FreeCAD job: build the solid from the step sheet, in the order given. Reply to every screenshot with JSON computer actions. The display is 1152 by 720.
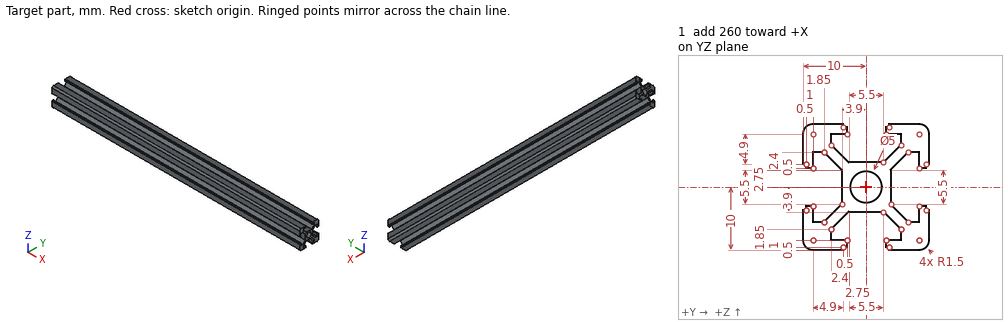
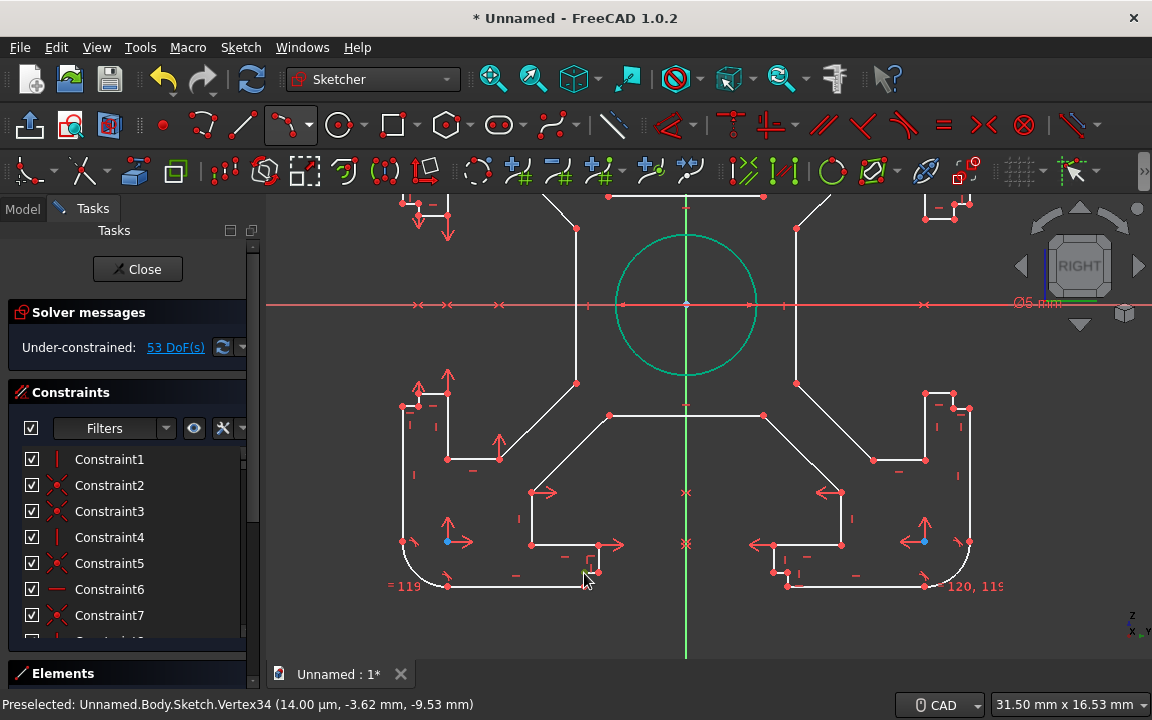
{"action": "left_click", "coordinate": [788, 573]}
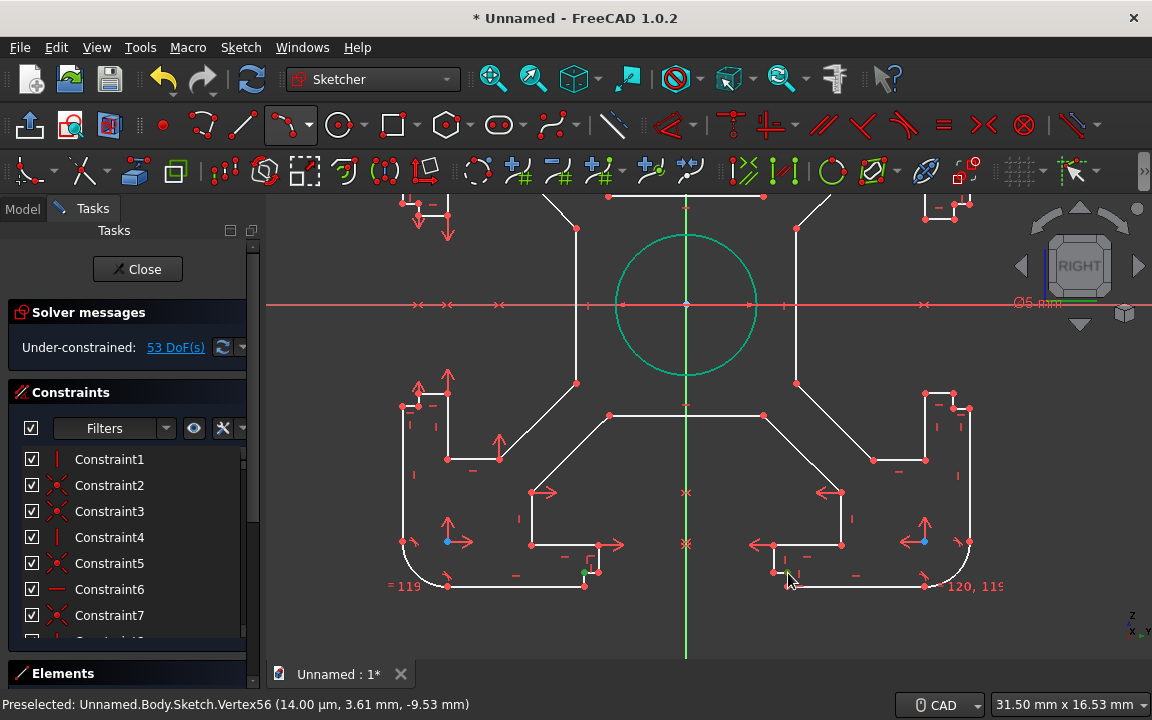
{"action": "left_click", "coordinate": [686, 602]}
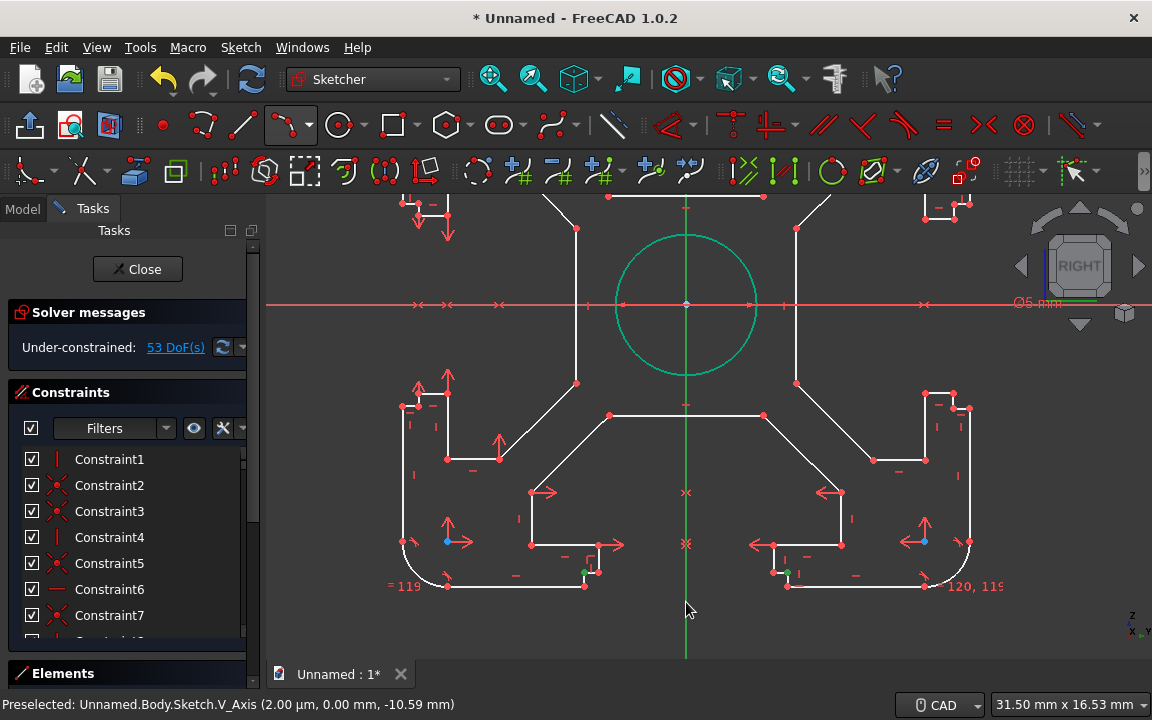
{"action": "key", "text": "s"}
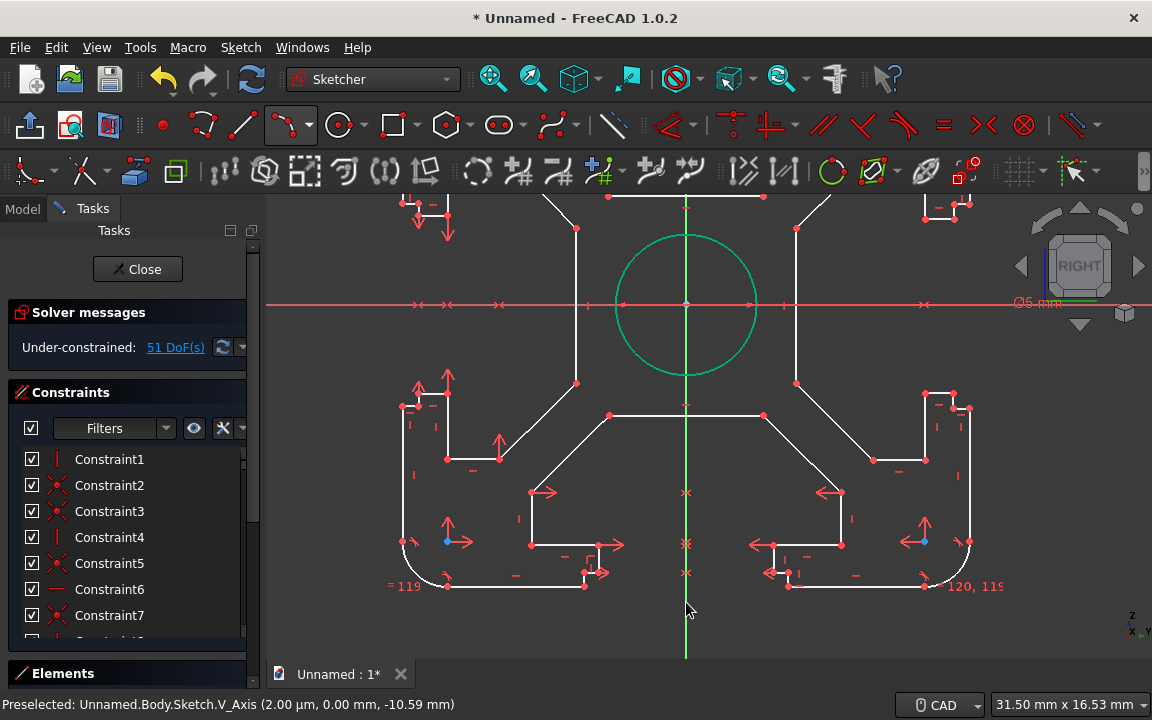
{"action": "left_click", "coordinate": [419, 406]}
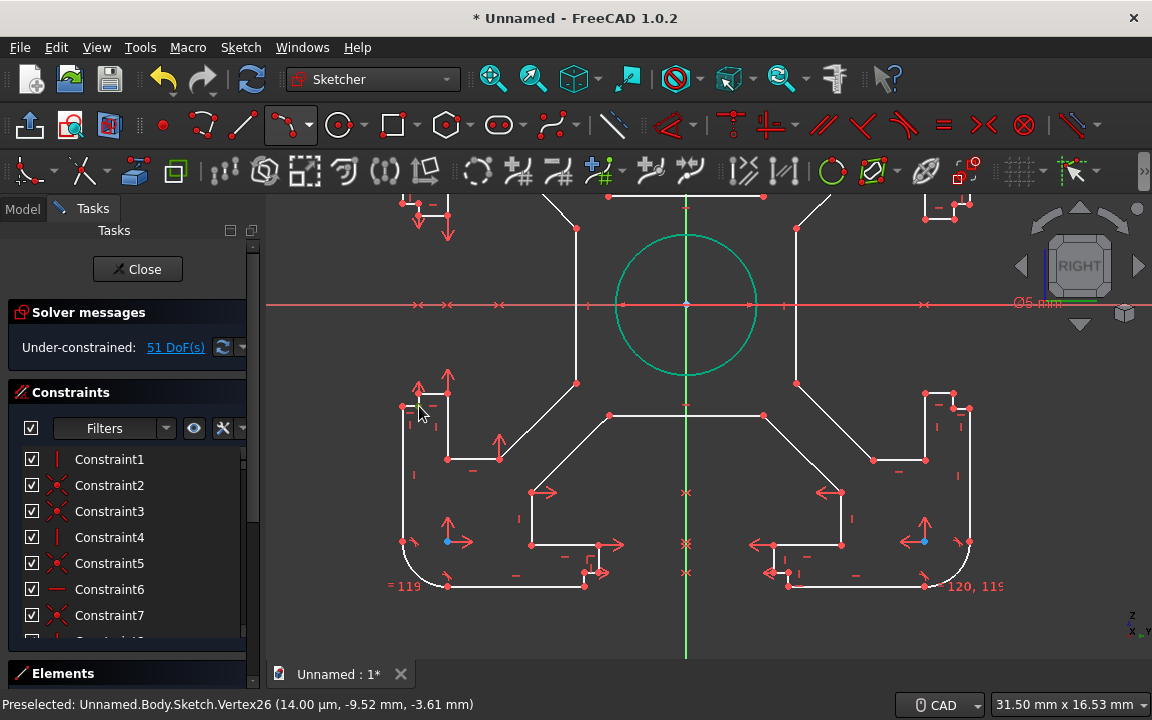
{"action": "left_click", "coordinate": [953, 409]}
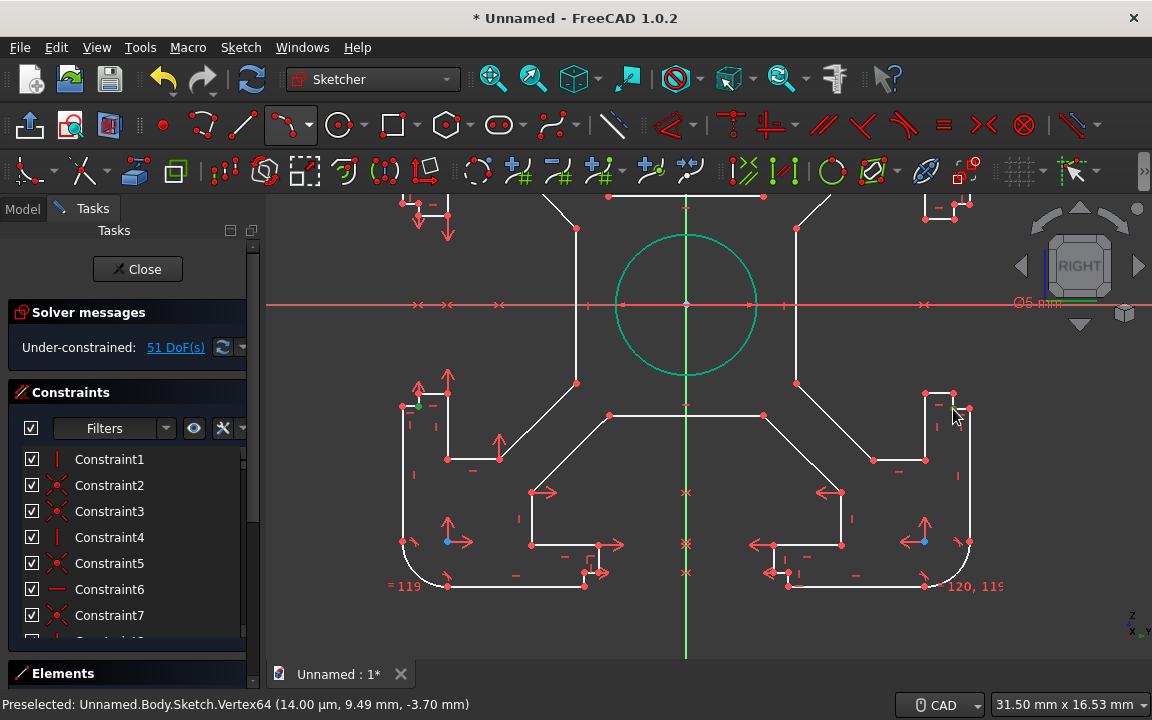
{"action": "left_click", "coordinate": [686, 602]}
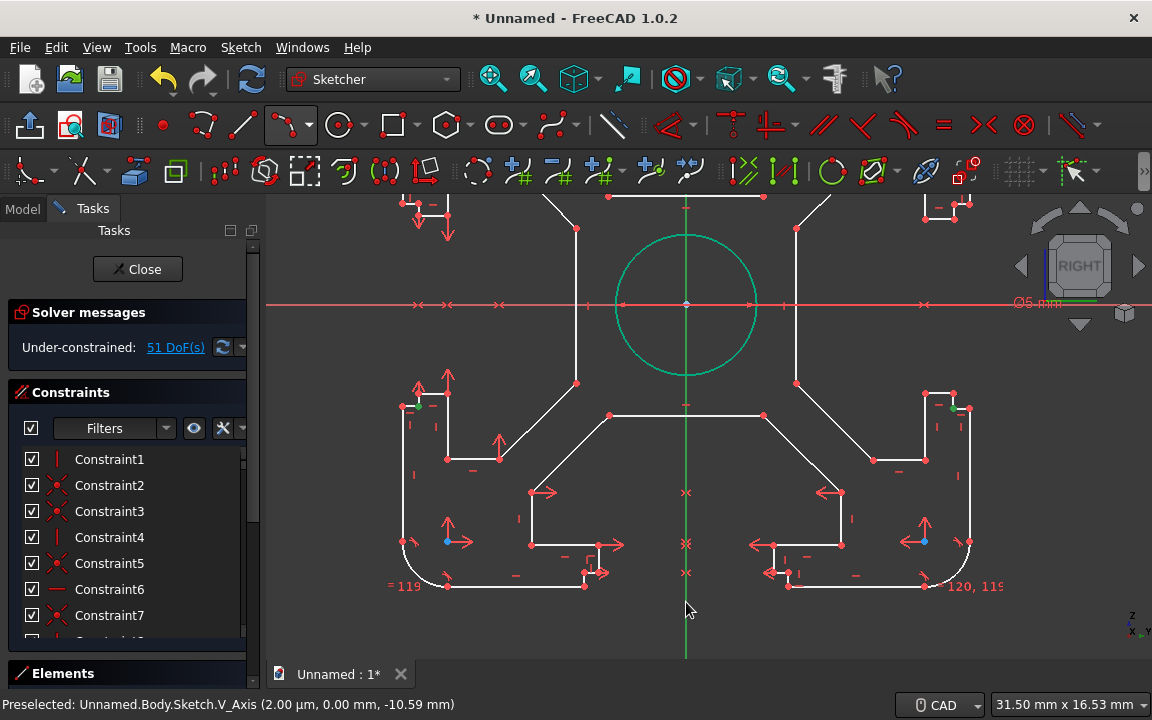
{"action": "left_click", "coordinate": [984, 126]}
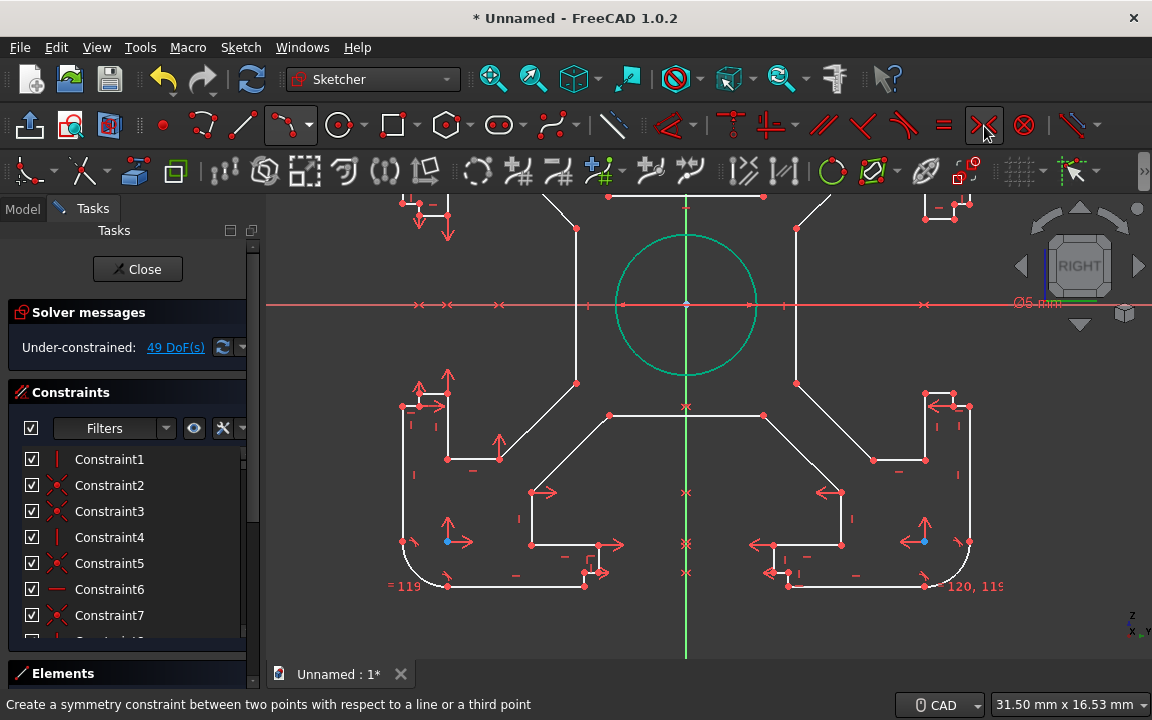
{"action": "left_click", "coordinate": [448, 394]}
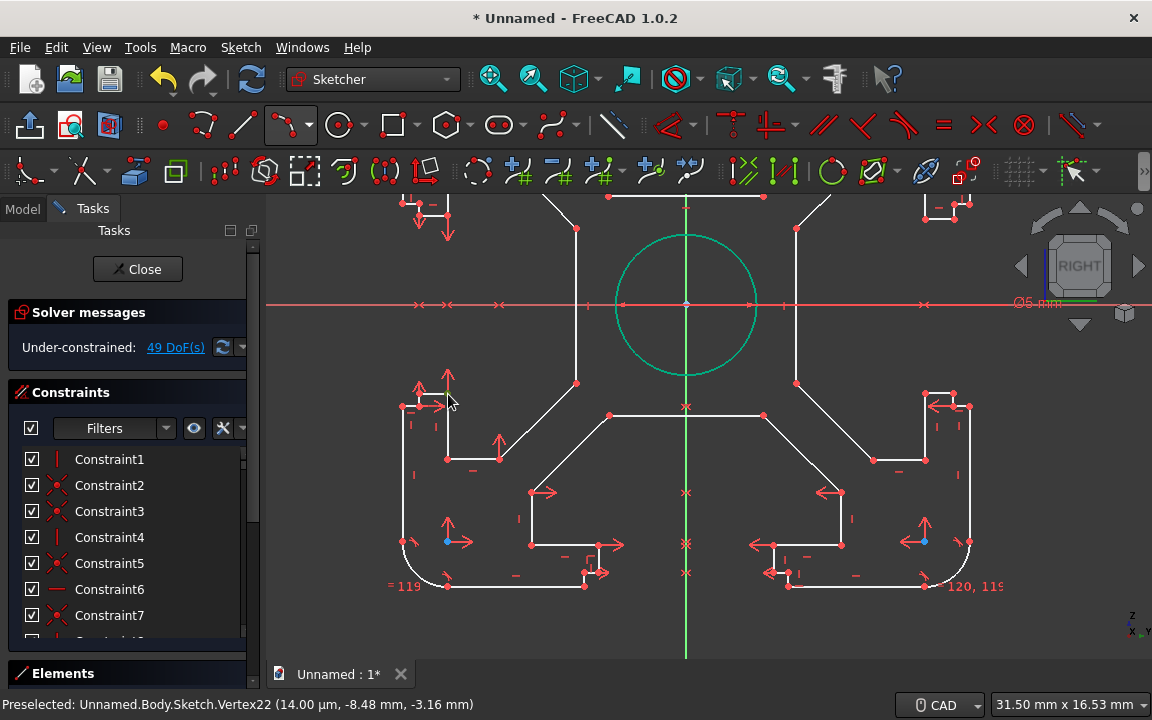
{"action": "left_click", "coordinate": [925, 393]}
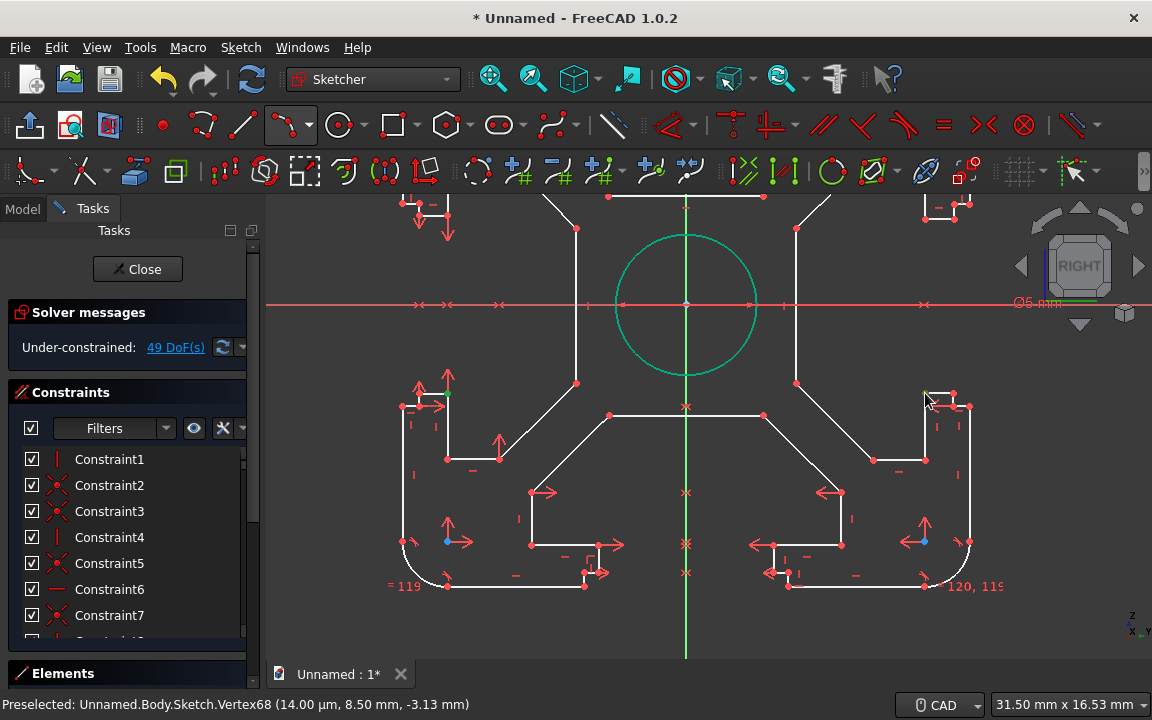
{"action": "left_click", "coordinate": [686, 602]}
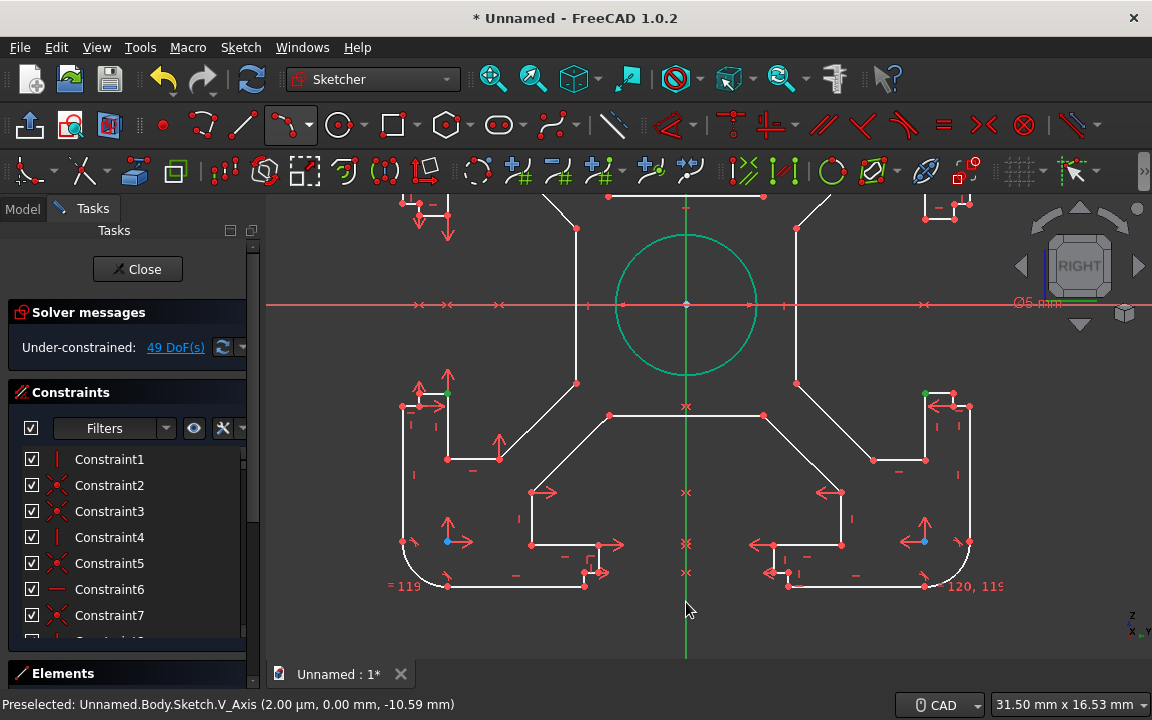
{"action": "key", "text": "s"}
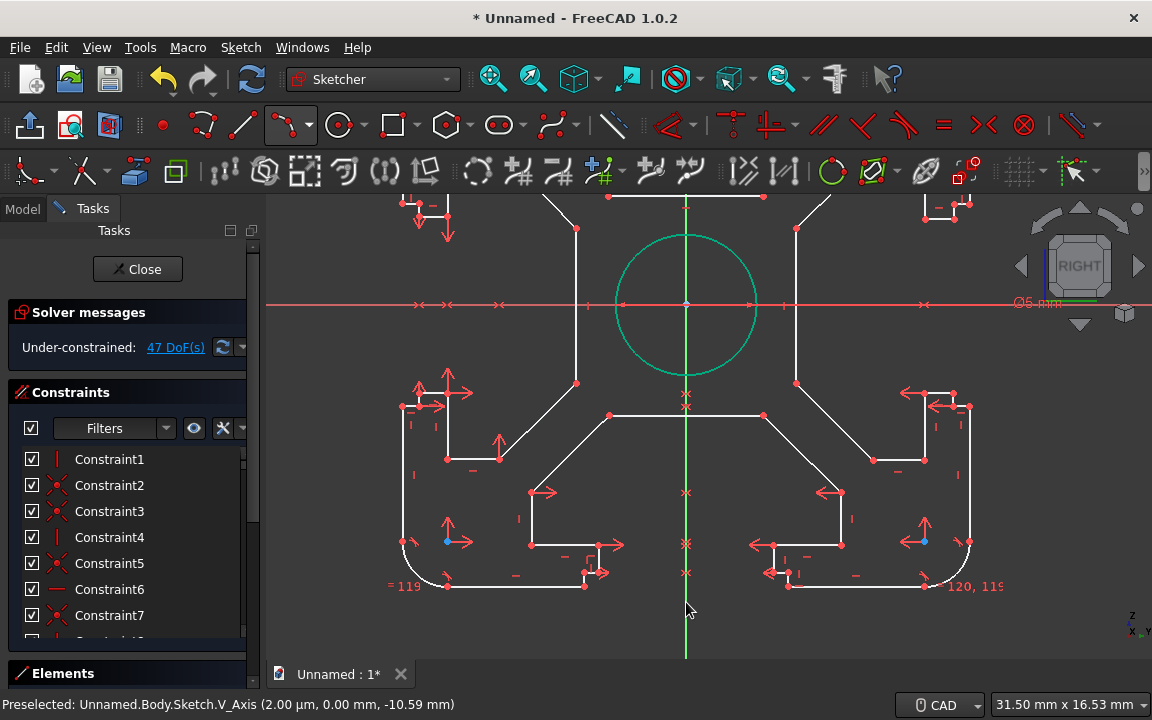
{"action": "left_click", "coordinate": [499, 459]}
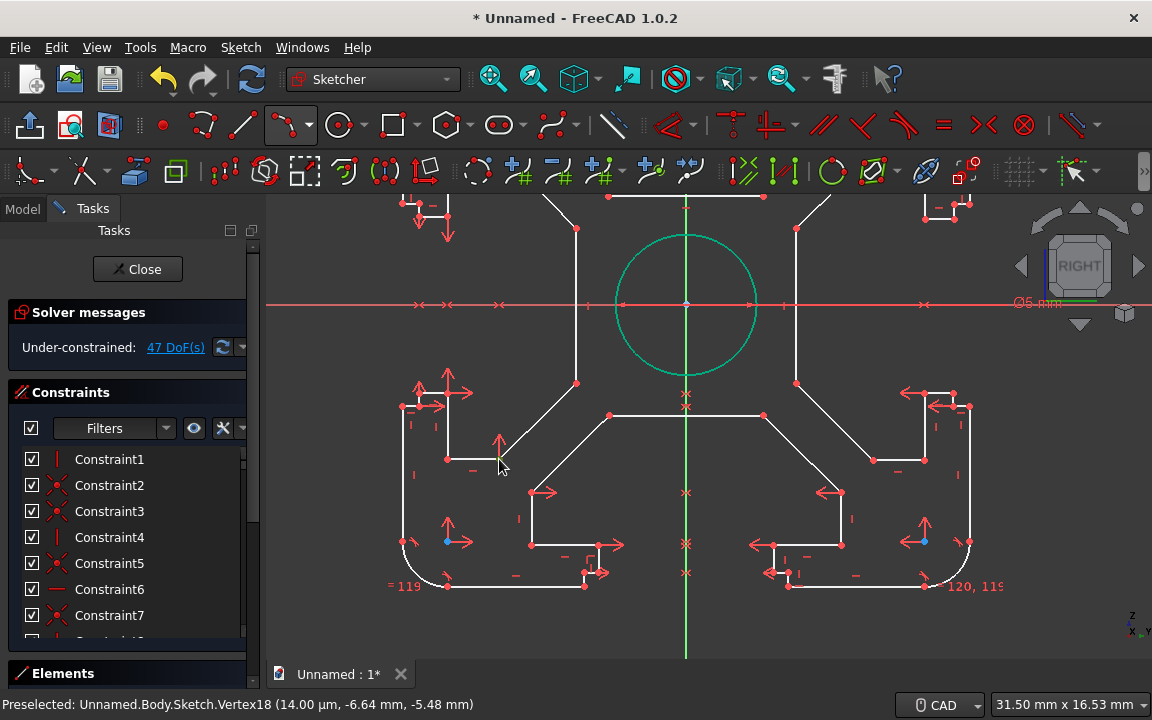
{"action": "left_click", "coordinate": [873, 460]}